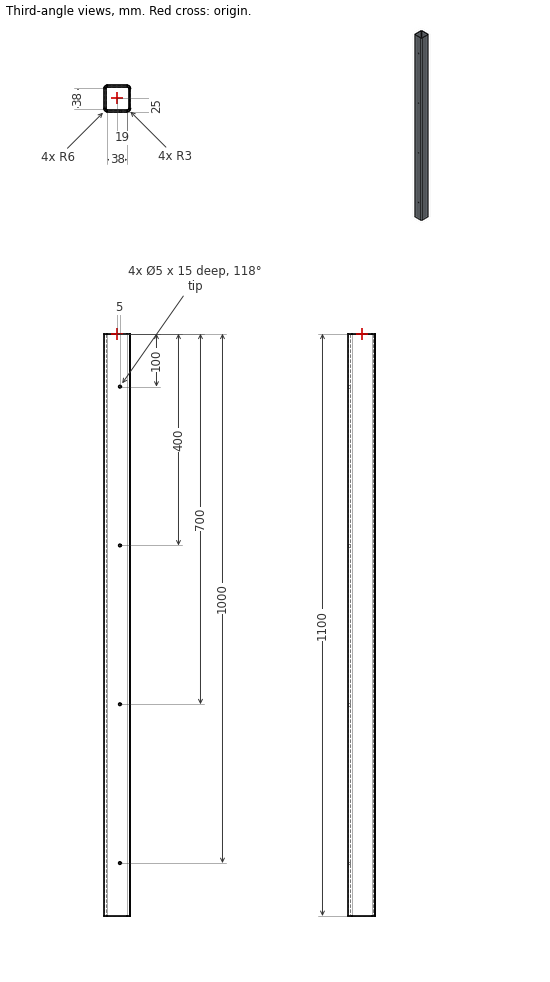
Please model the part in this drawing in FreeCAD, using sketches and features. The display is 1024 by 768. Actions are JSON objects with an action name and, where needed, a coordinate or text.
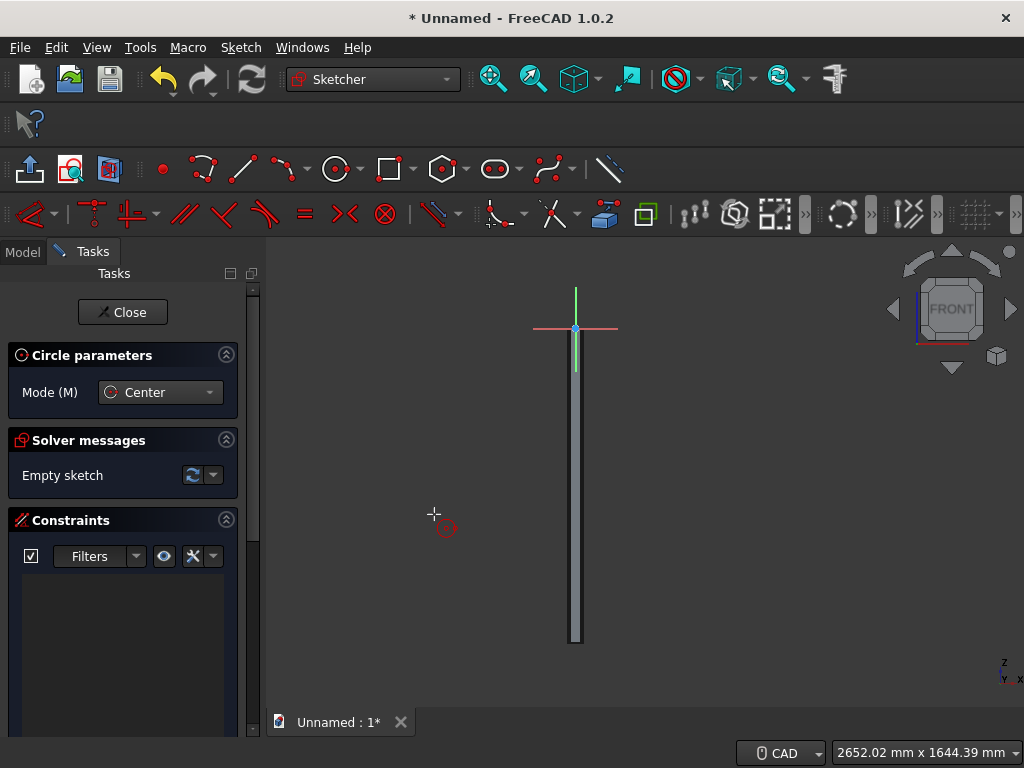
{"action": "scroll", "coordinate": [577, 357], "scroll_direction": "up", "scroll_amount": 18}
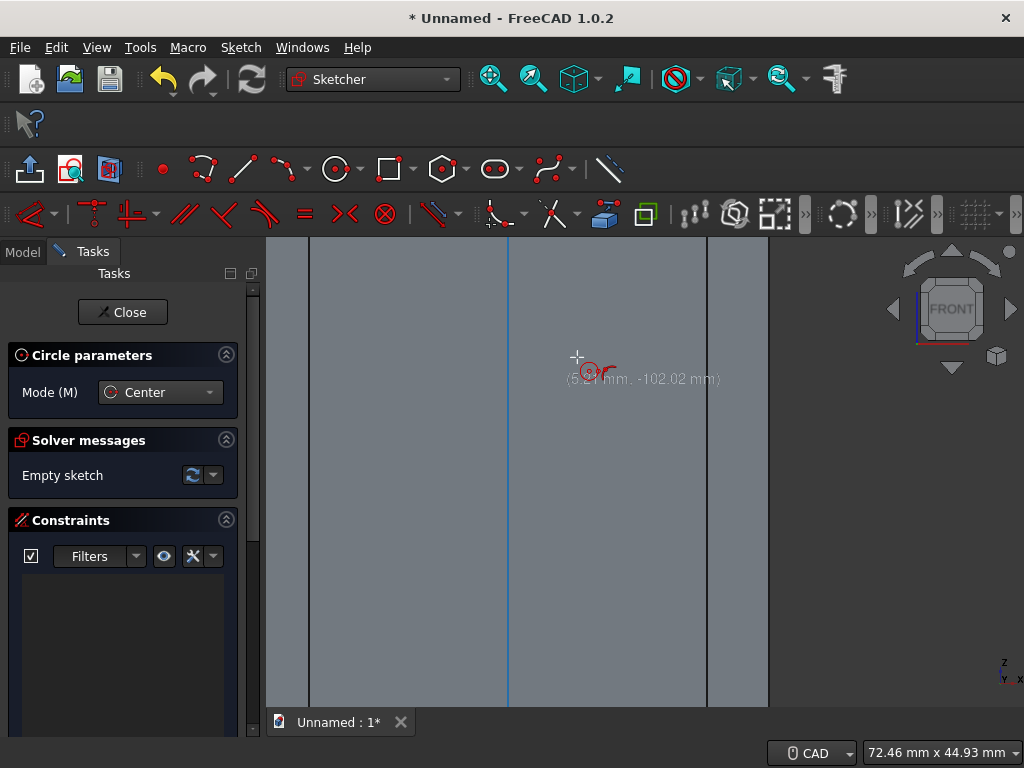
{"action": "scroll", "coordinate": [578, 331], "scroll_direction": "down", "scroll_amount": 17}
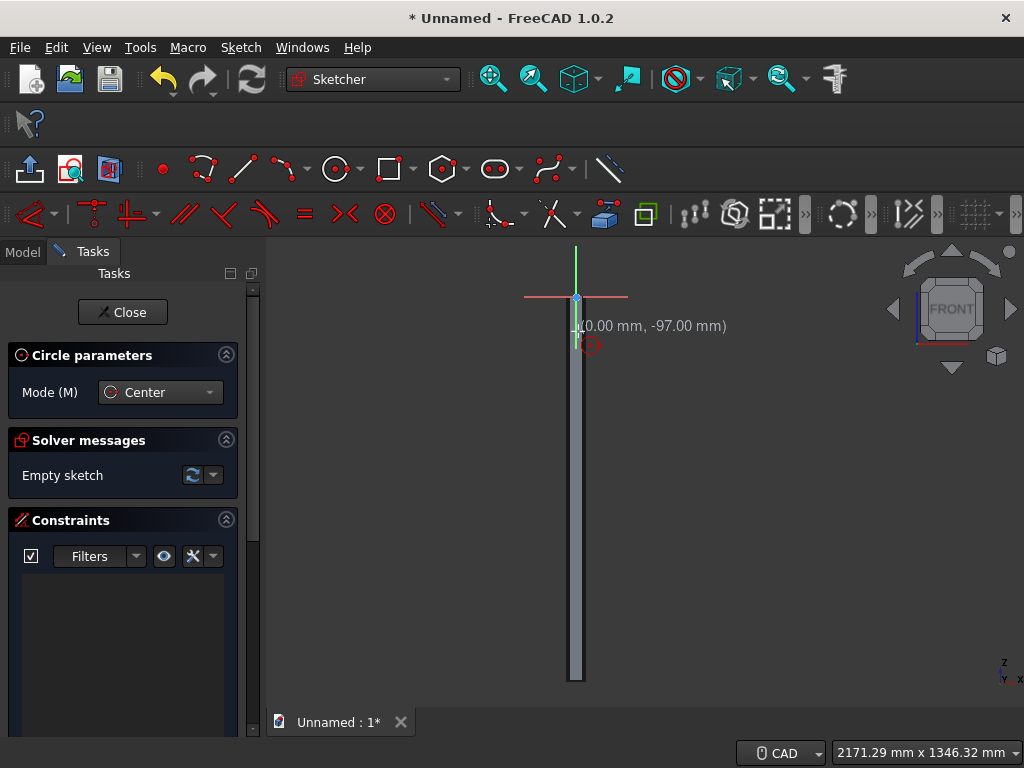
{"action": "scroll", "coordinate": [578, 332], "scroll_direction": "up", "scroll_amount": 12}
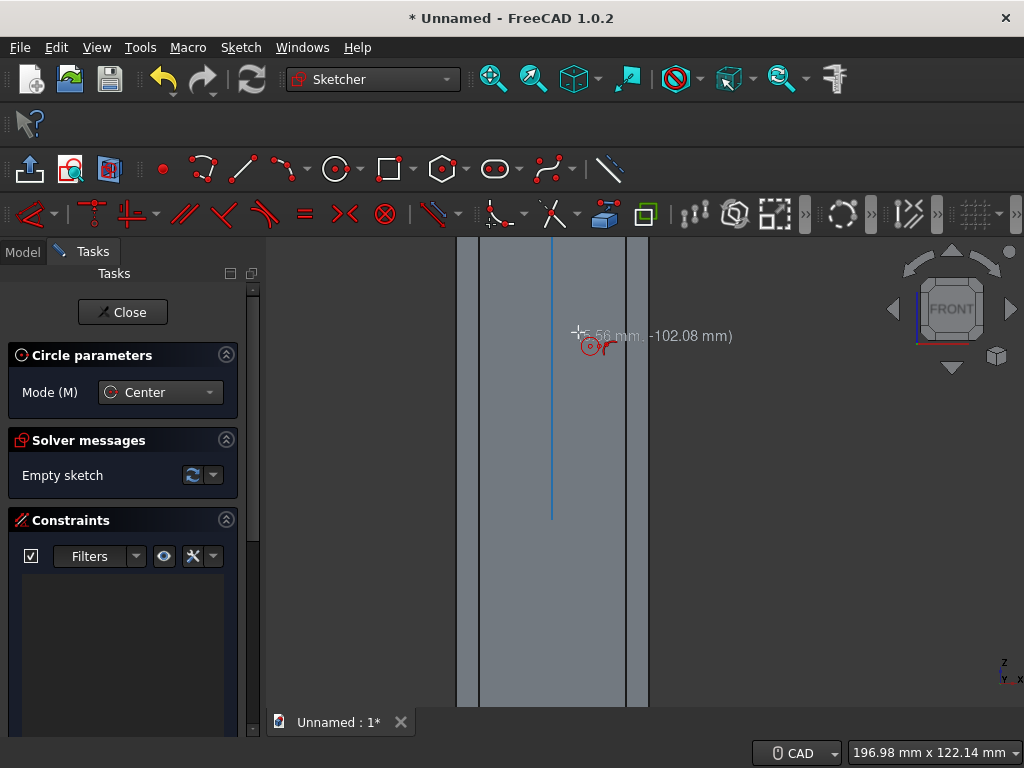
{"action": "left_click", "coordinate": [572, 333]}
{"action": "mouse_move", "coordinate": [579, 326]}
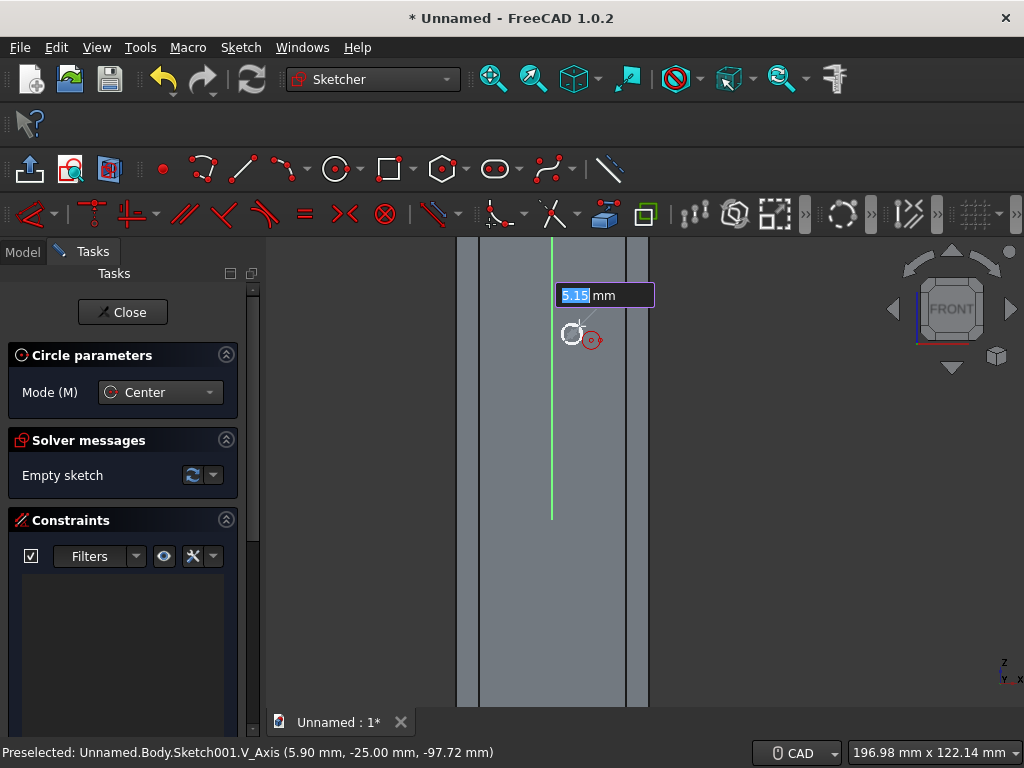
{"action": "type", "text": "5"}
{"action": "key", "text": "Return"}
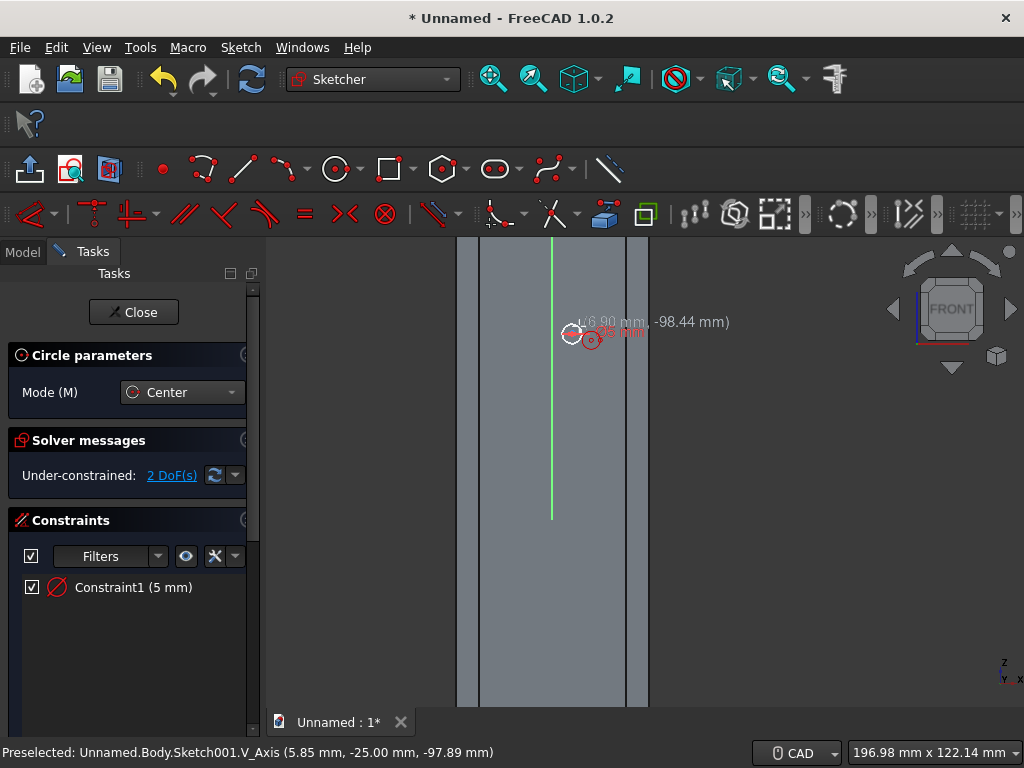
{"action": "scroll", "coordinate": [577, 359], "scroll_direction": "down", "scroll_amount": 13}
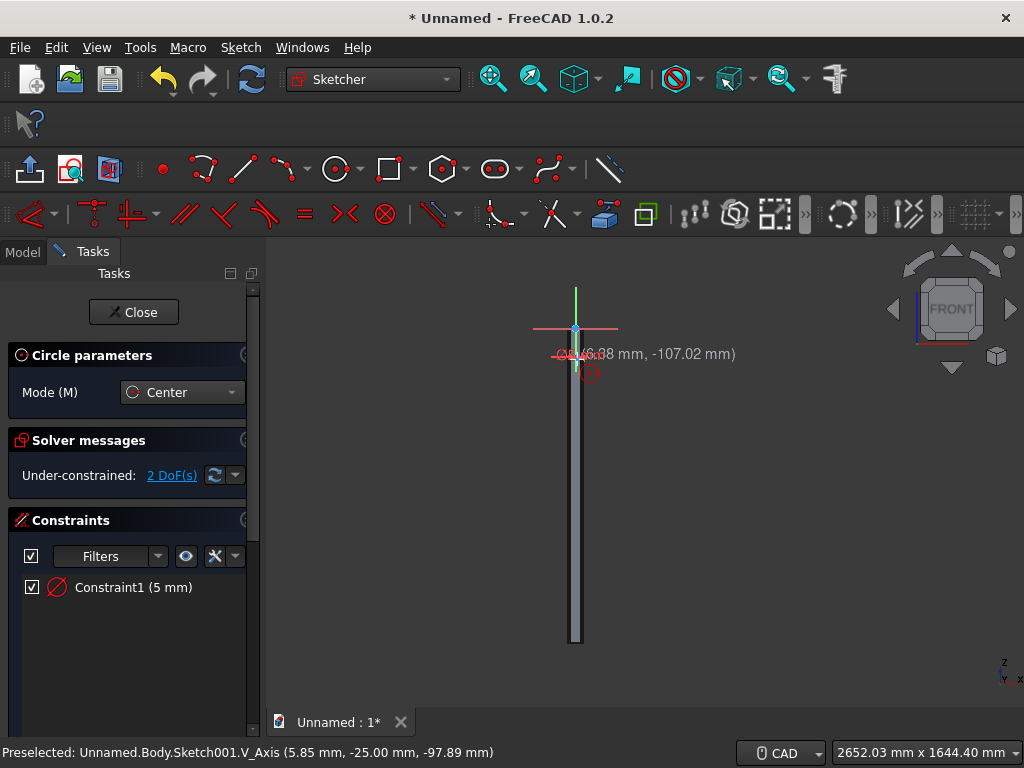
{"action": "scroll", "coordinate": [577, 443], "scroll_direction": "up", "scroll_amount": 18}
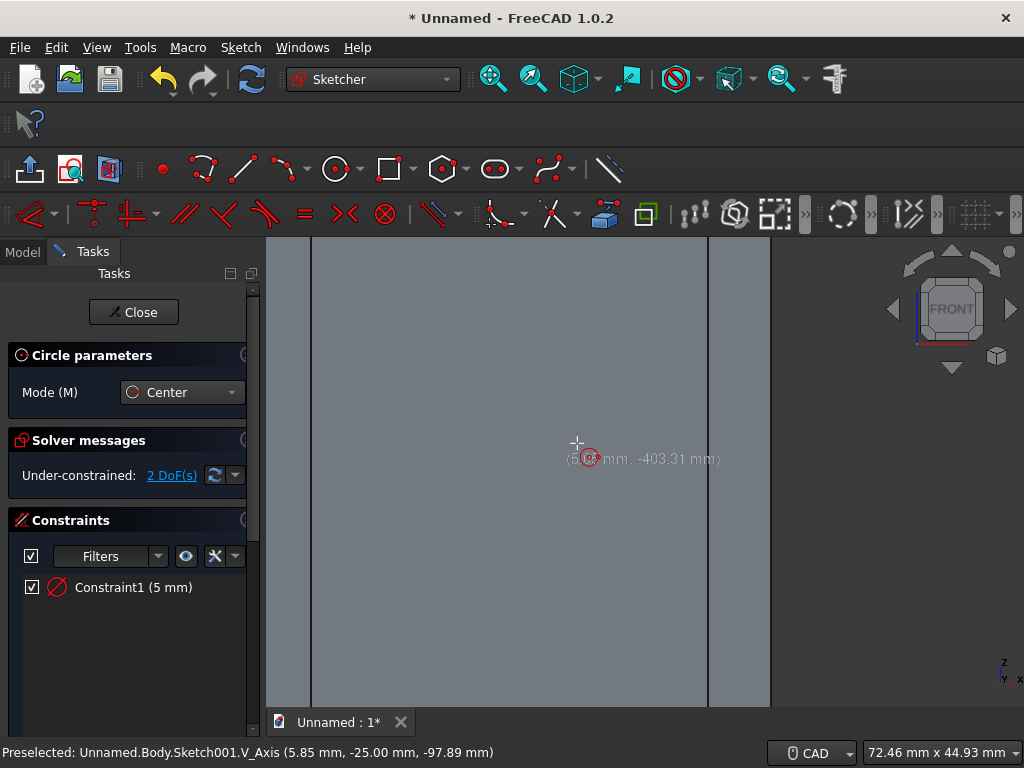
{"action": "scroll", "coordinate": [577, 437], "scroll_direction": "down", "scroll_amount": 17}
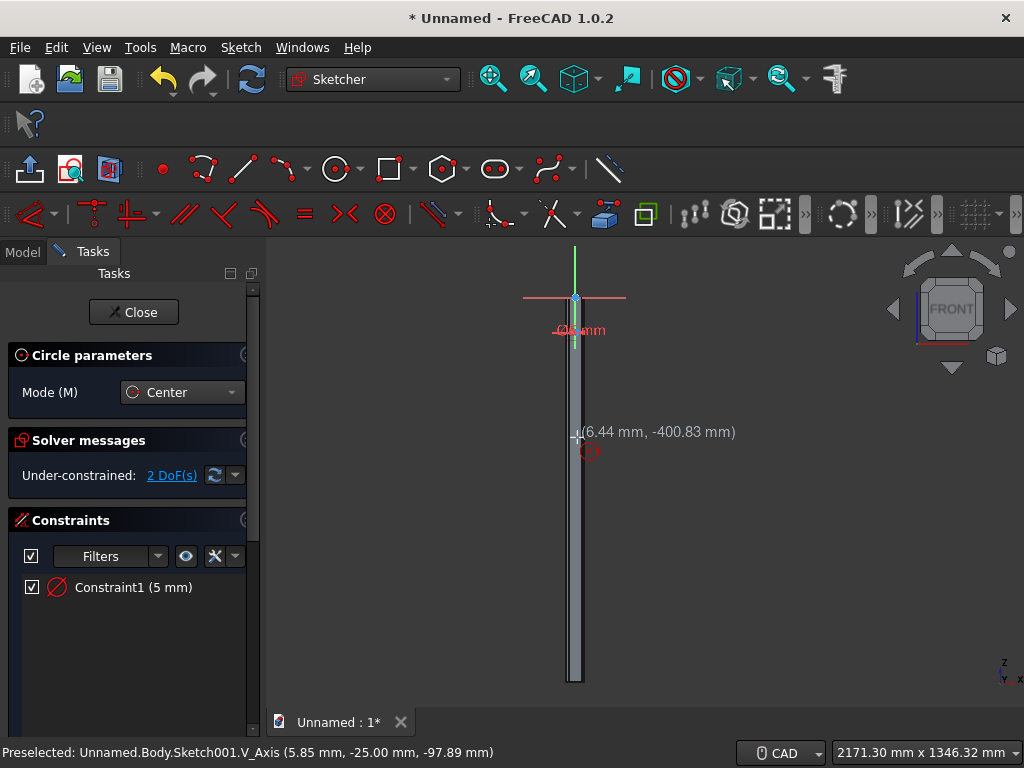
{"action": "scroll", "coordinate": [577, 437], "scroll_direction": "up", "scroll_amount": 12}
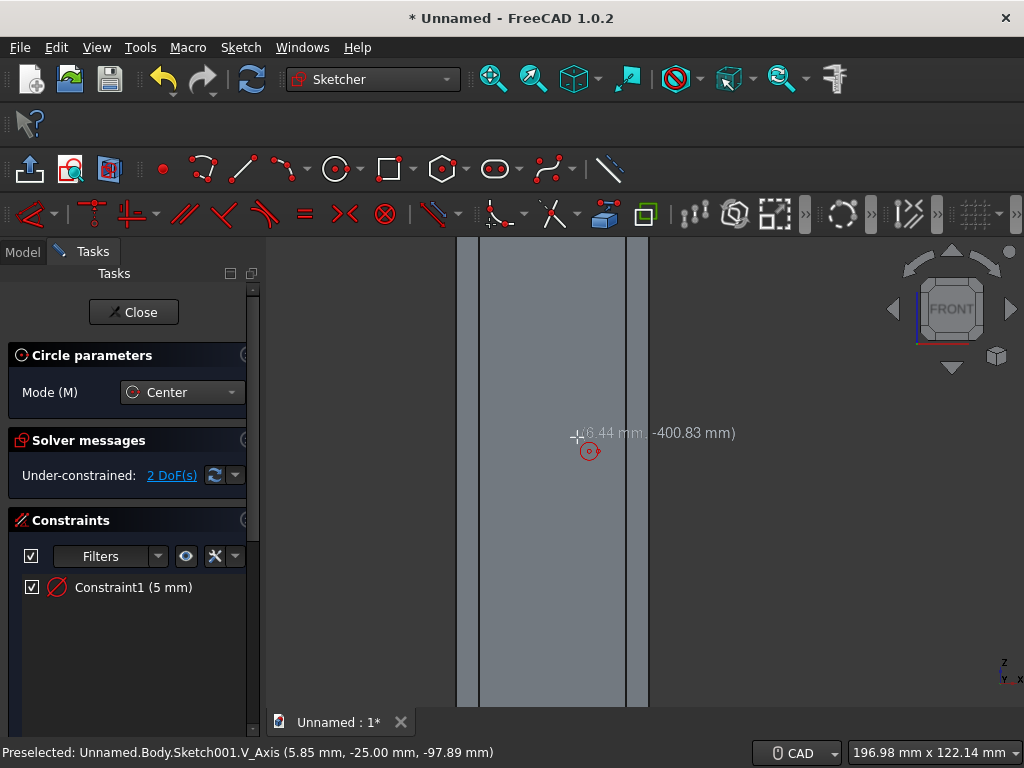
{"action": "left_click", "coordinate": [572, 434]}
{"action": "mouse_move", "coordinate": [579, 428]}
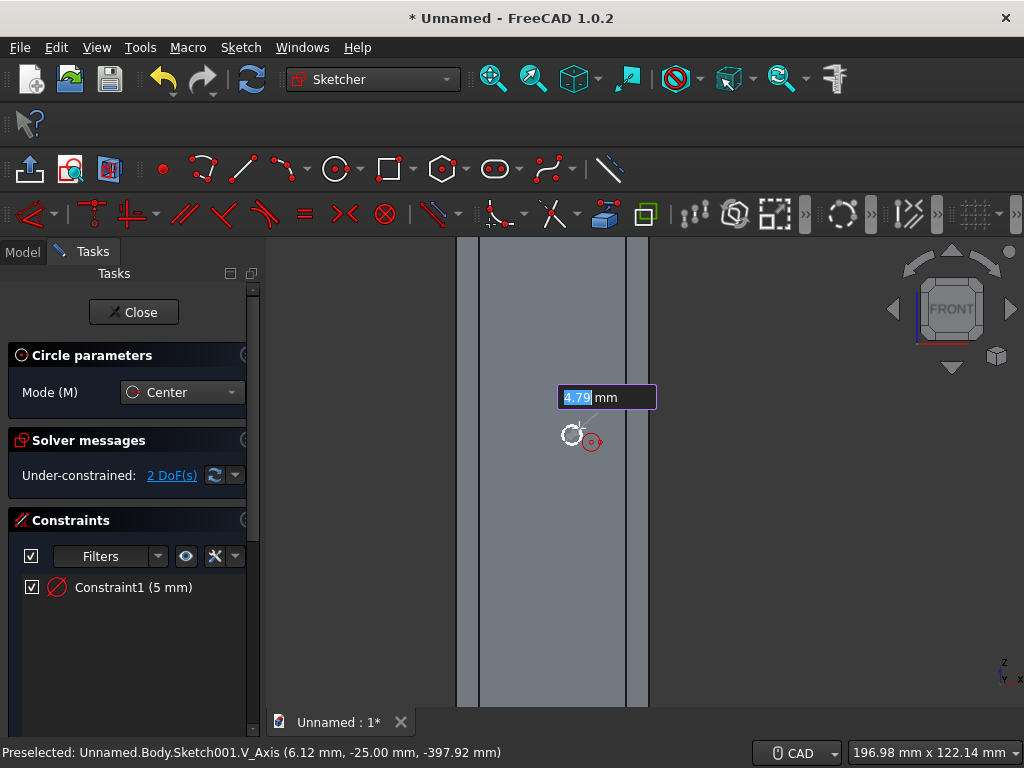
{"action": "type", "text": "5"}
{"action": "key", "text": "Return"}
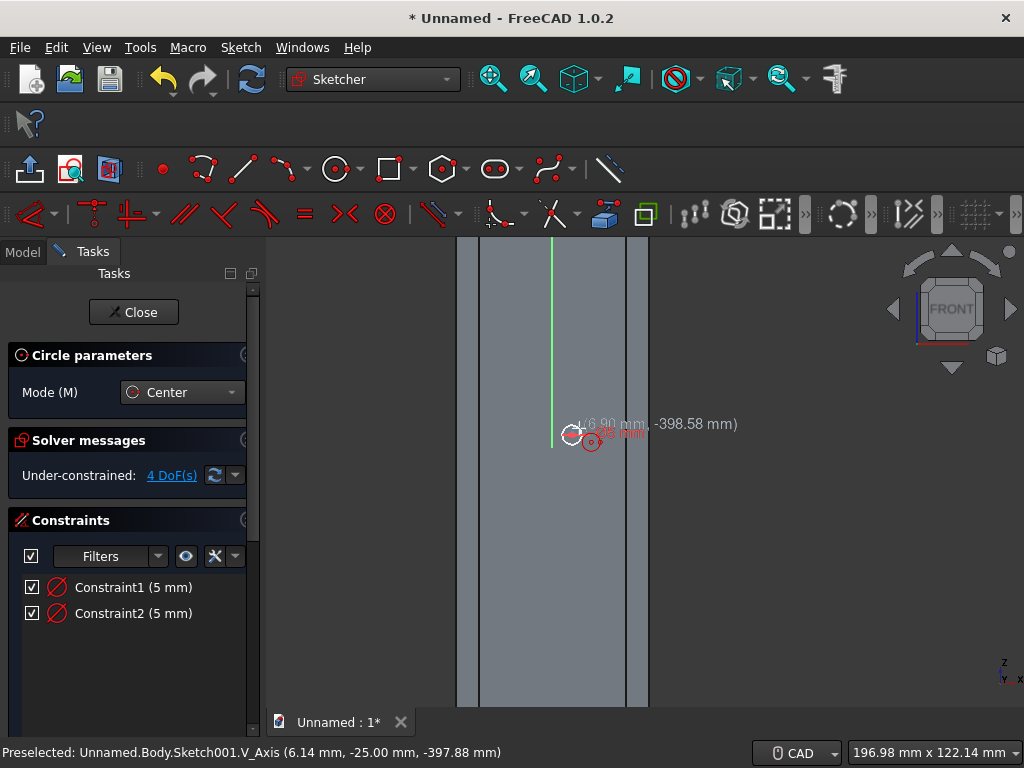
{"action": "scroll", "coordinate": [577, 444], "scroll_direction": "down", "scroll_amount": 13}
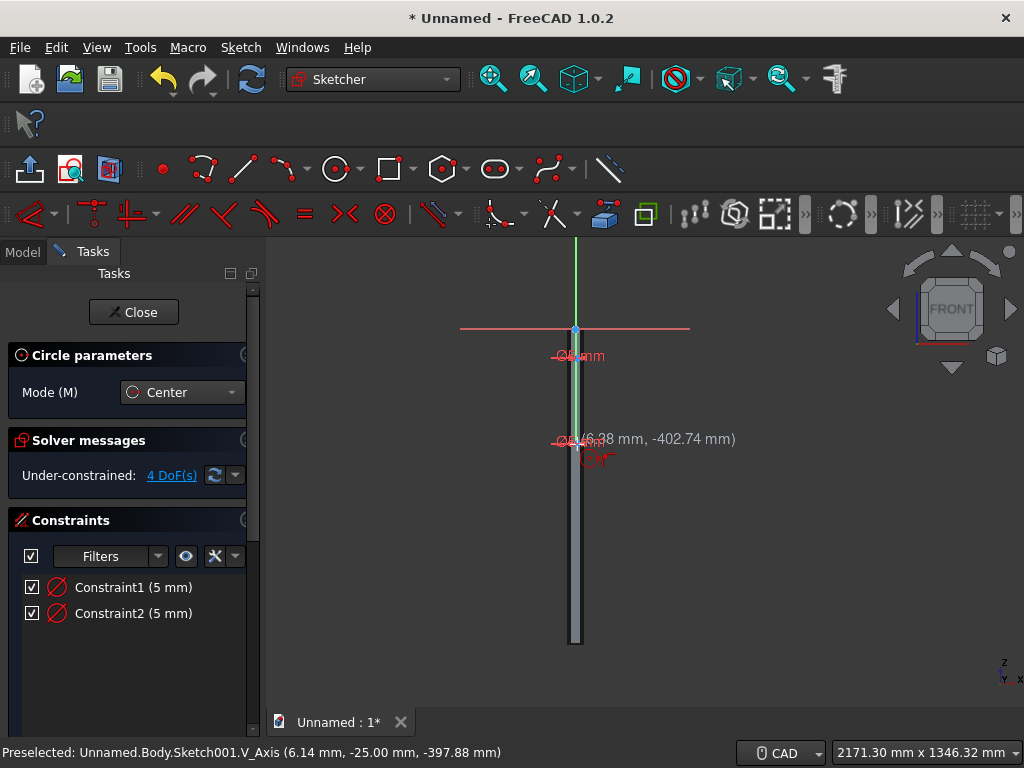
{"action": "scroll", "coordinate": [577, 529], "scroll_direction": "up", "scroll_amount": 18}